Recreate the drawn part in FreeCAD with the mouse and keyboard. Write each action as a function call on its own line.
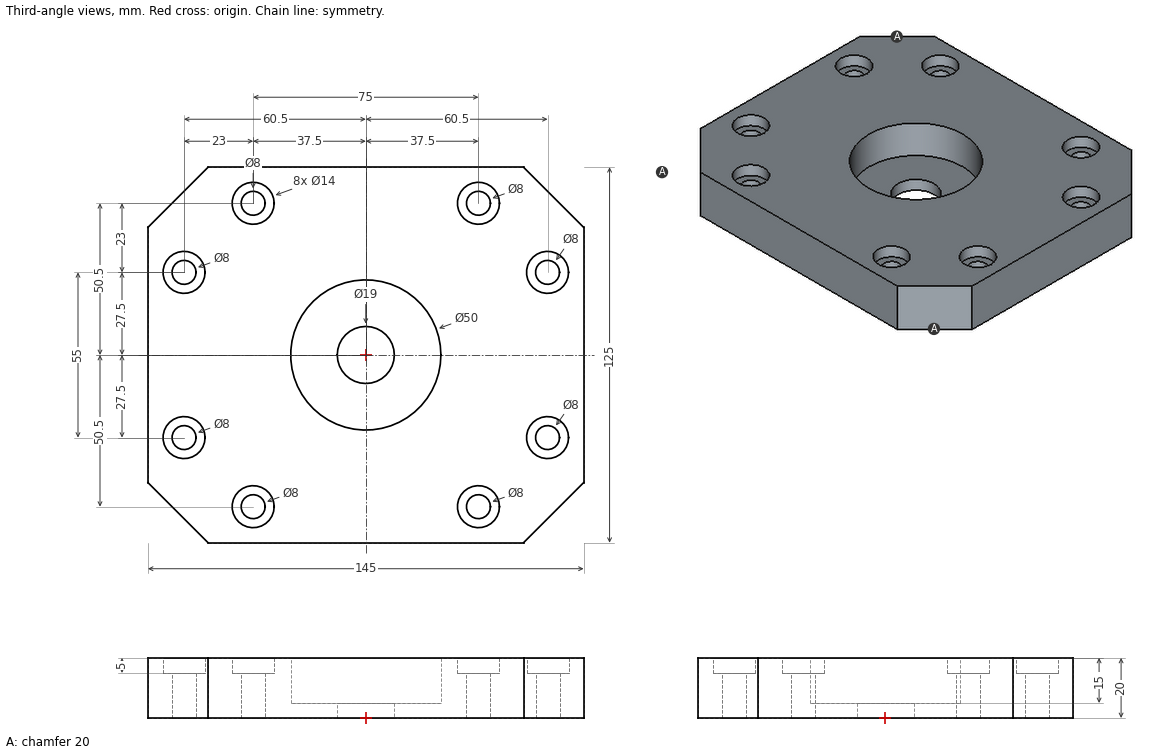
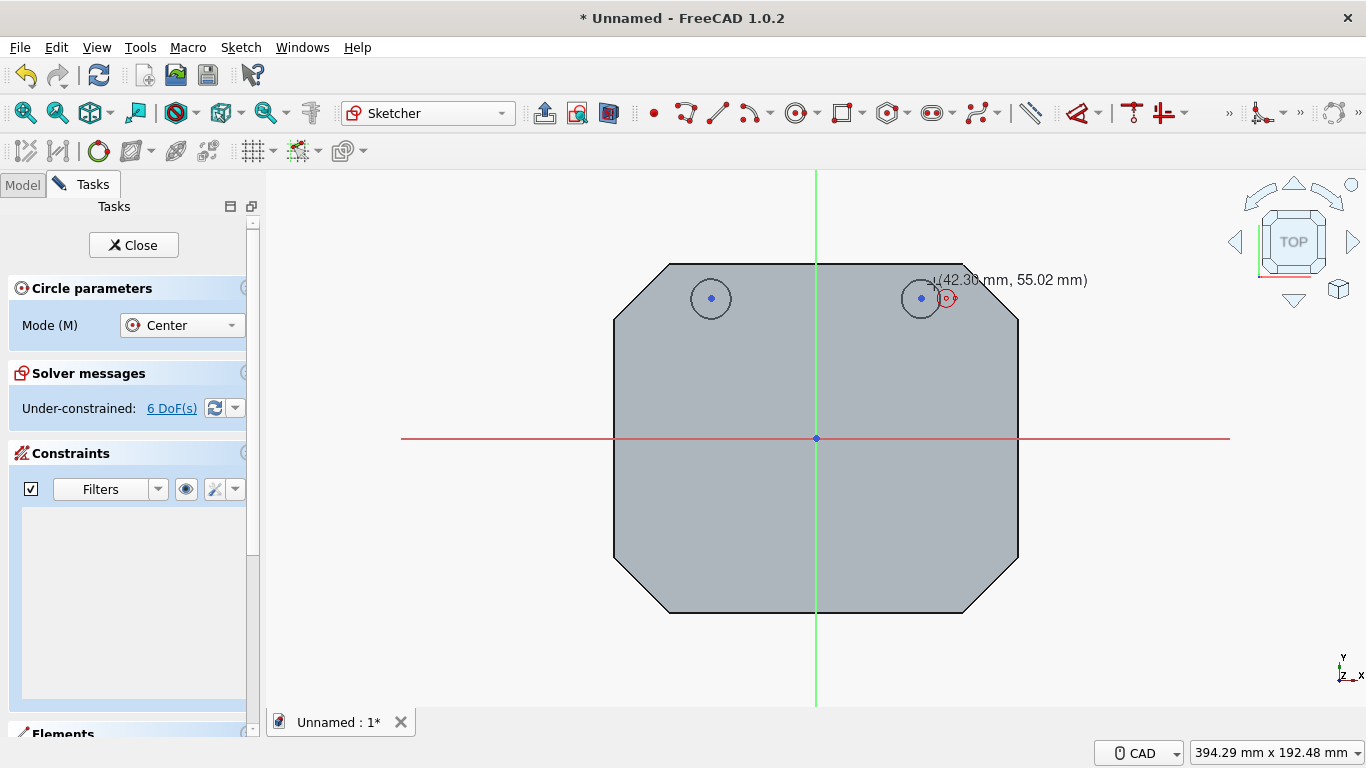
click(647, 362)
click(661, 348)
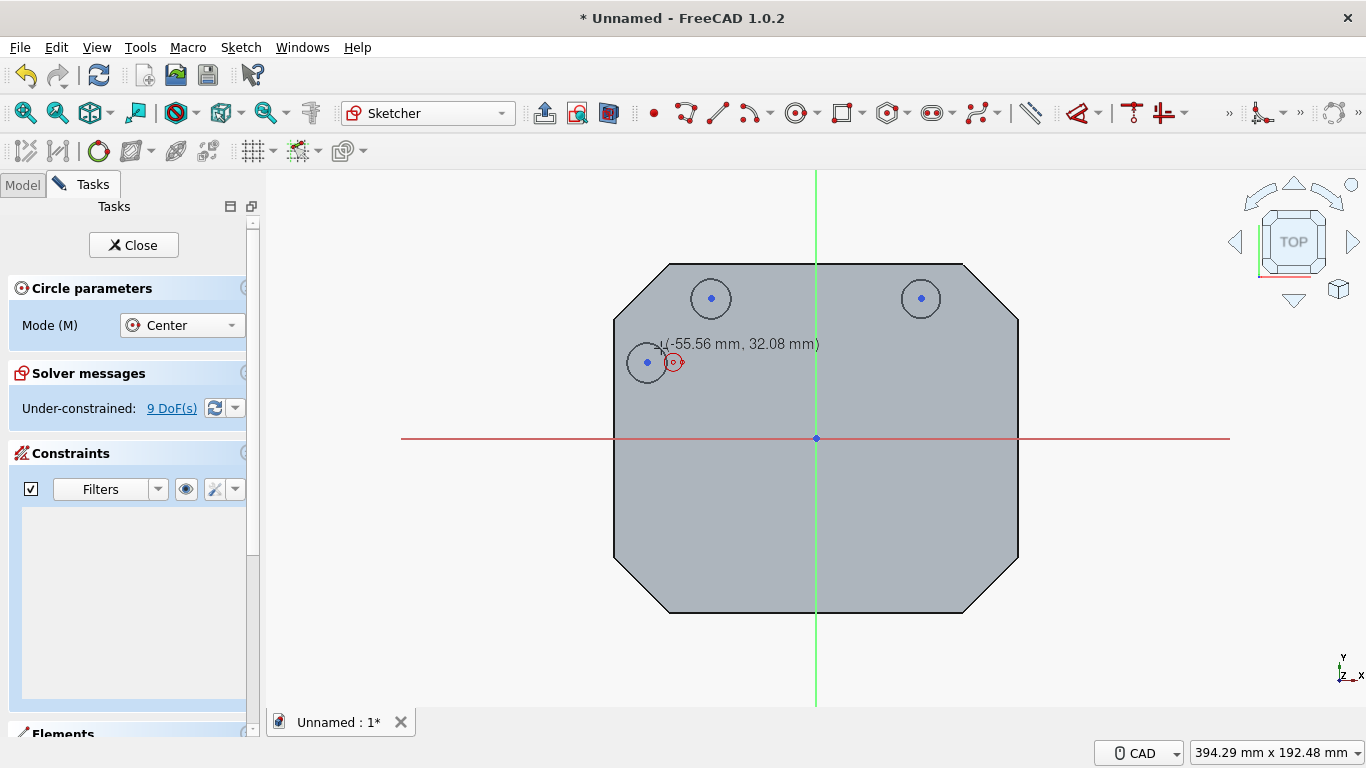
click(647, 515)
click(661, 501)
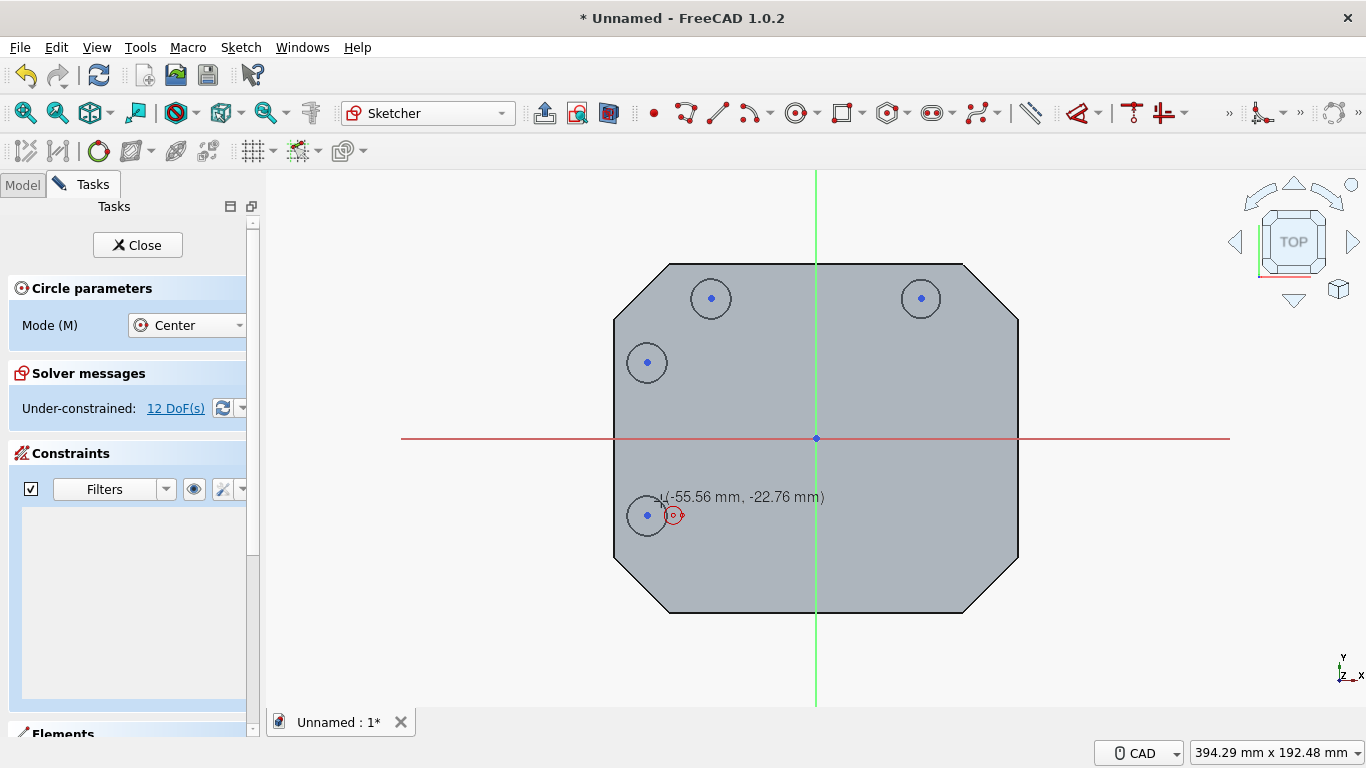
click(711, 579)
click(725, 566)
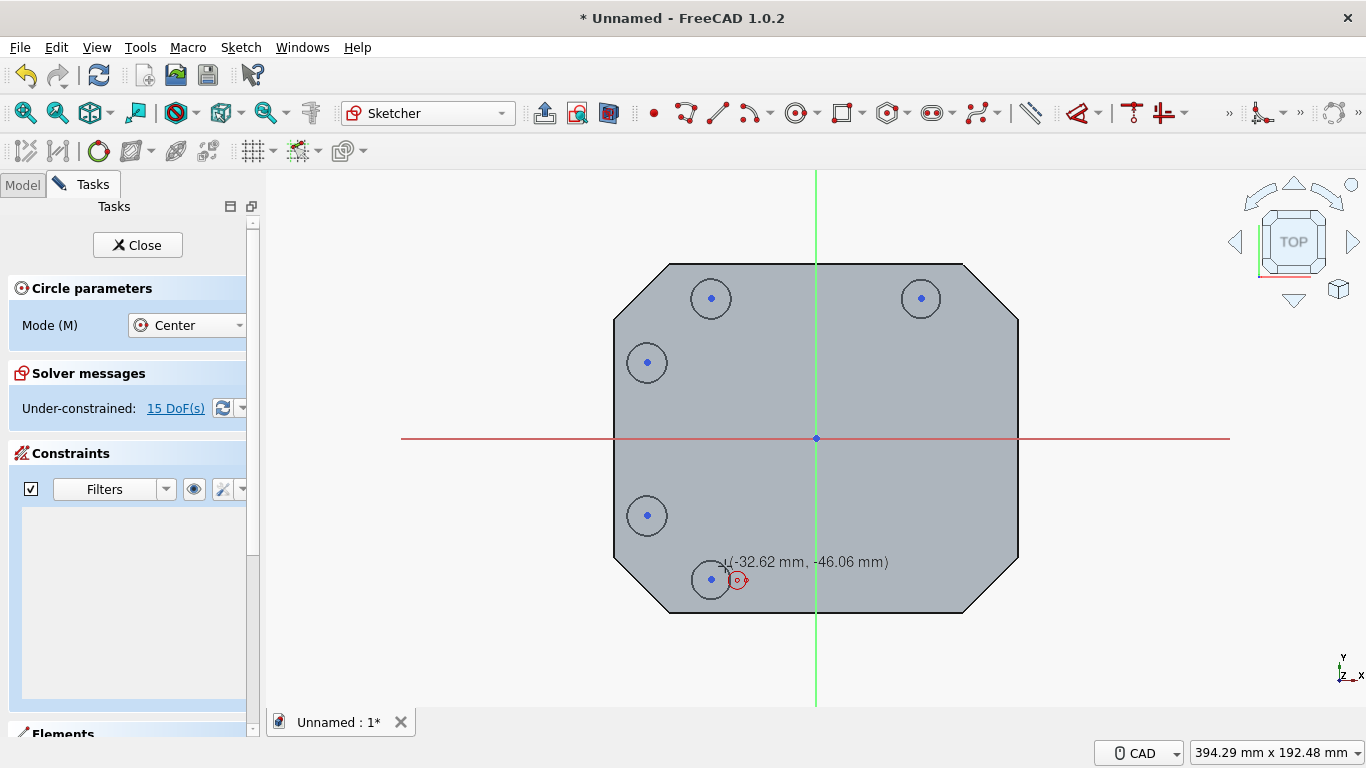
click(921, 579)
click(934, 566)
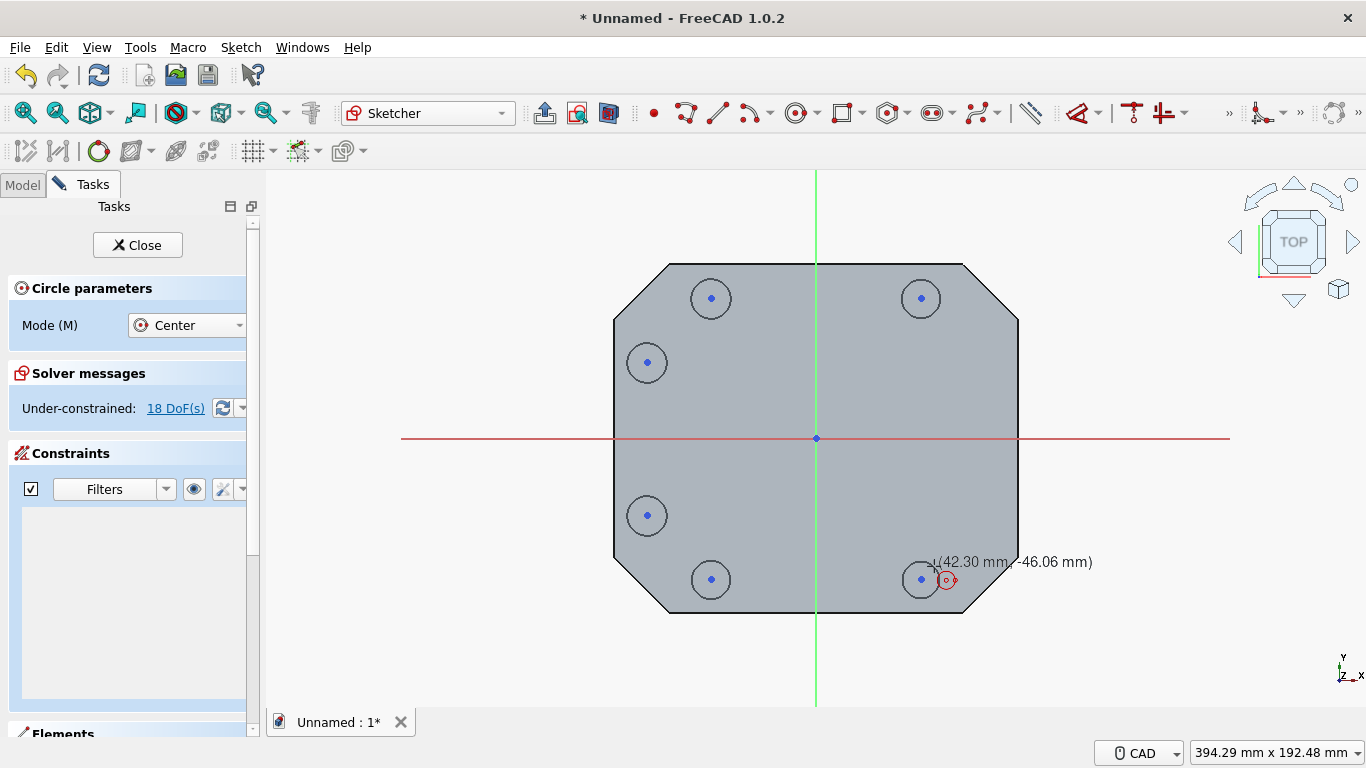
click(985, 362)
click(999, 348)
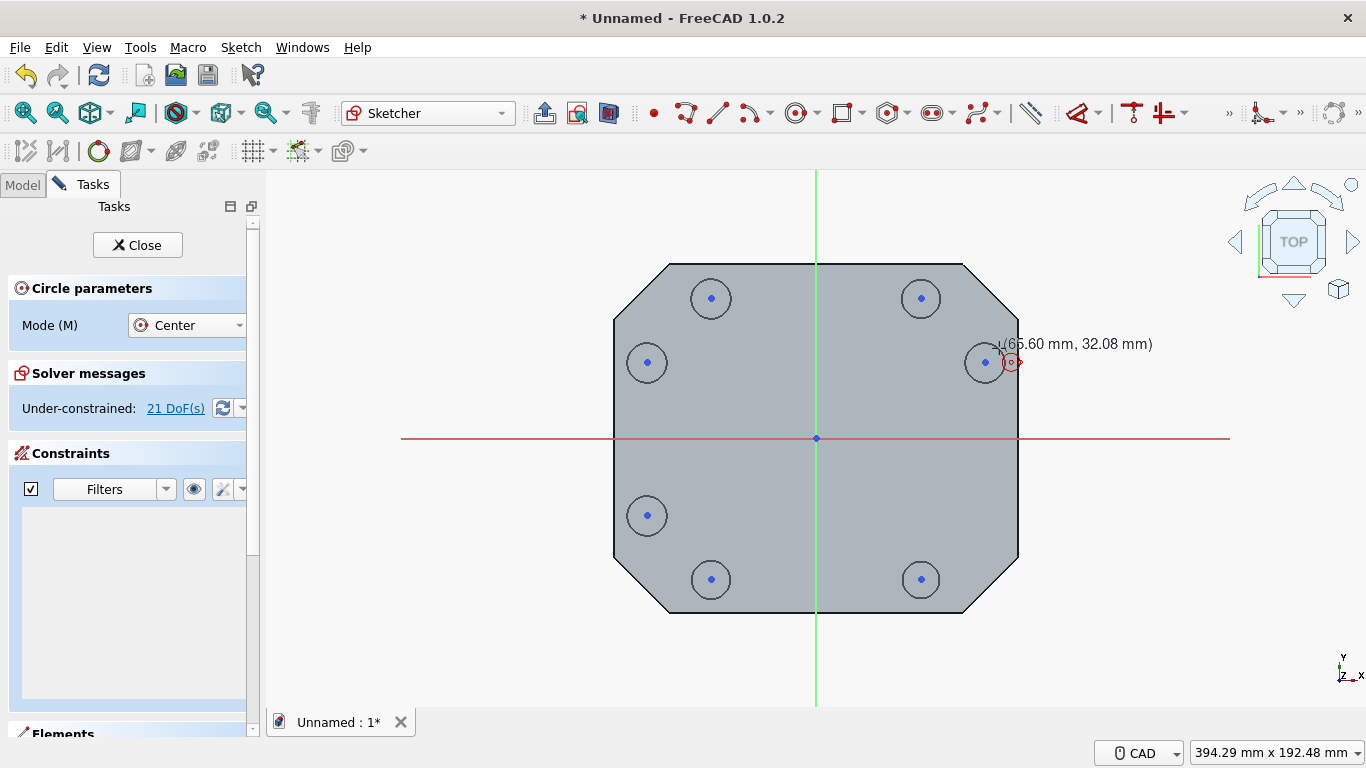
click(985, 515)
click(999, 501)
key(Escape)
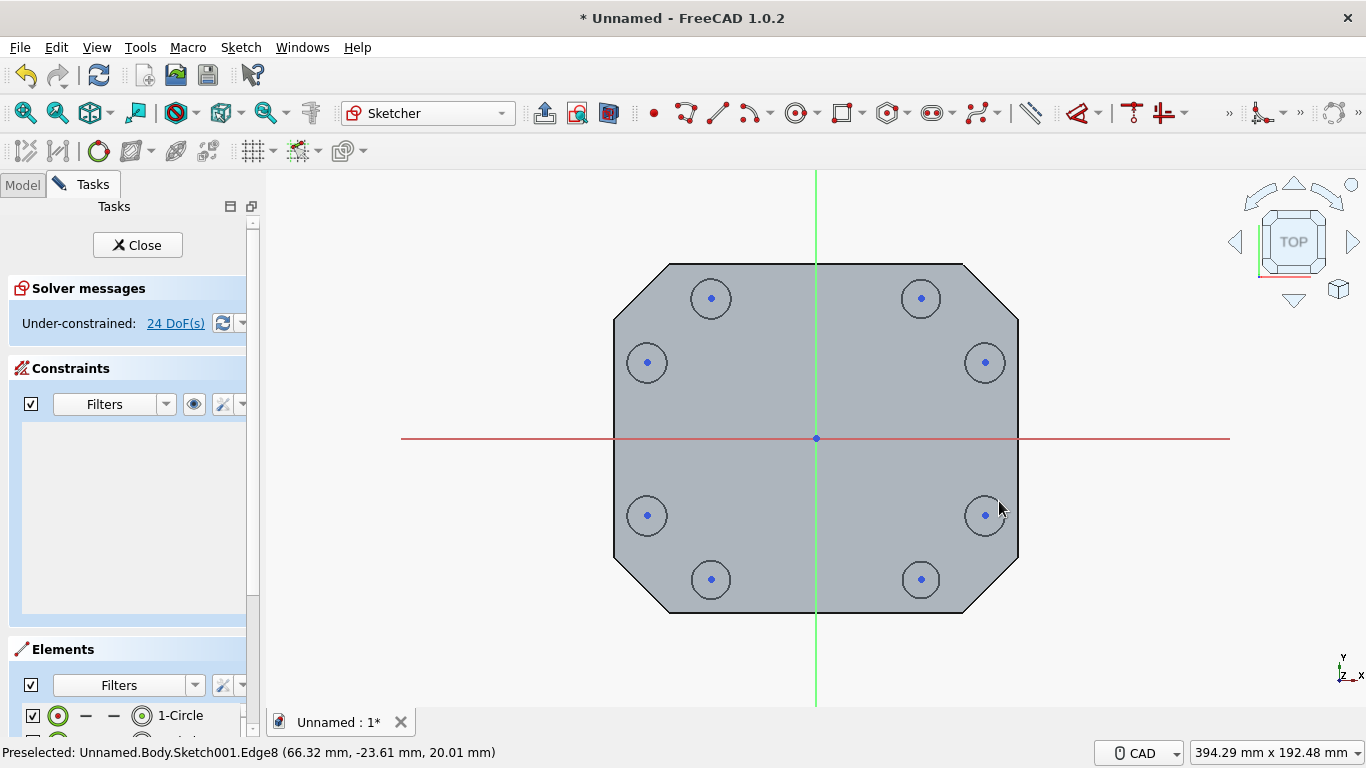
click(725, 285)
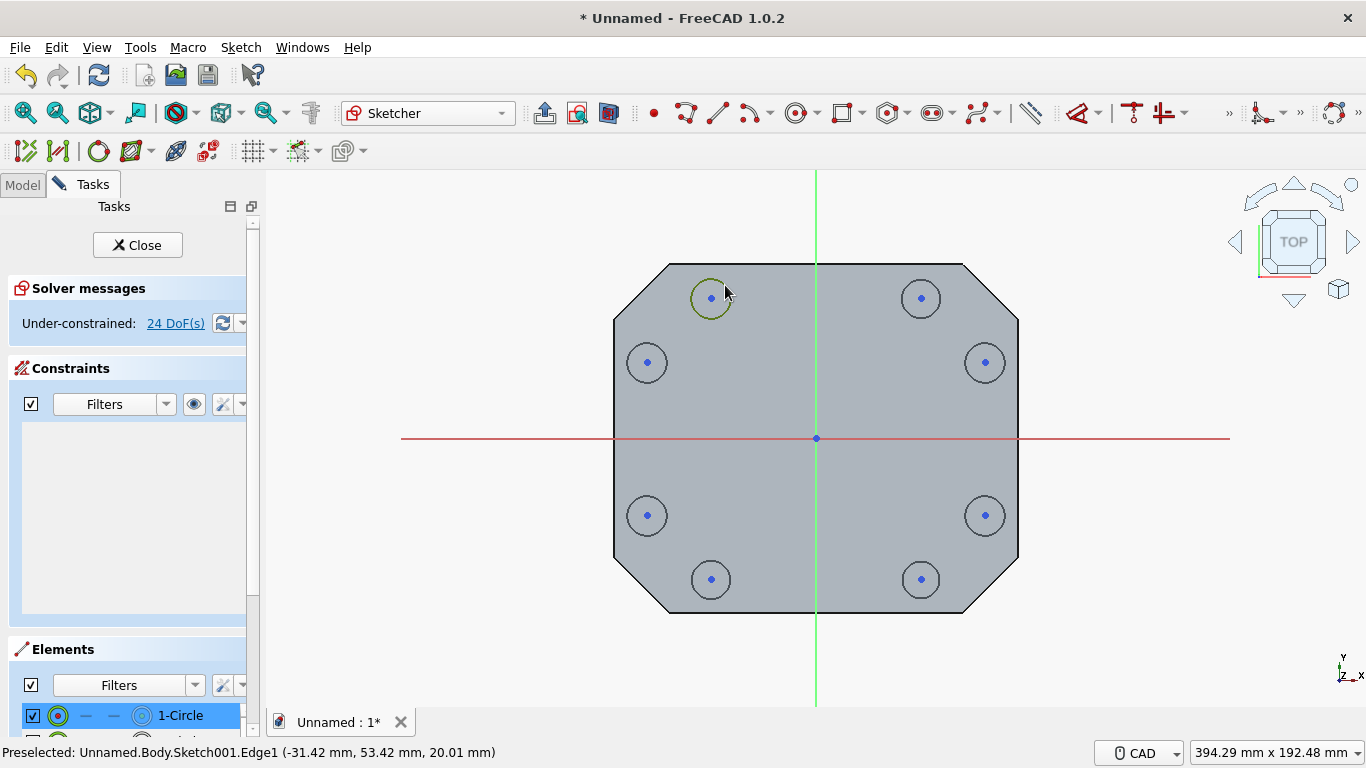
click(934, 285)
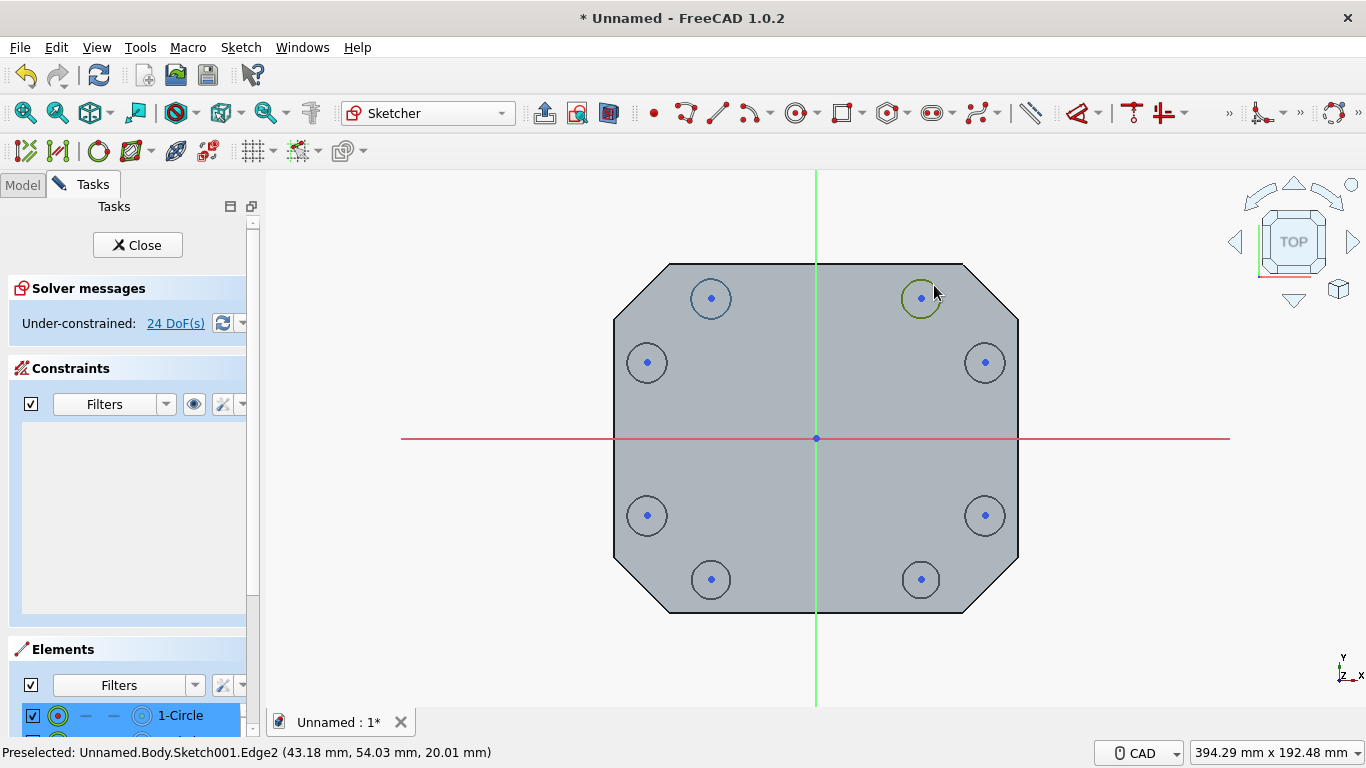
click(661, 349)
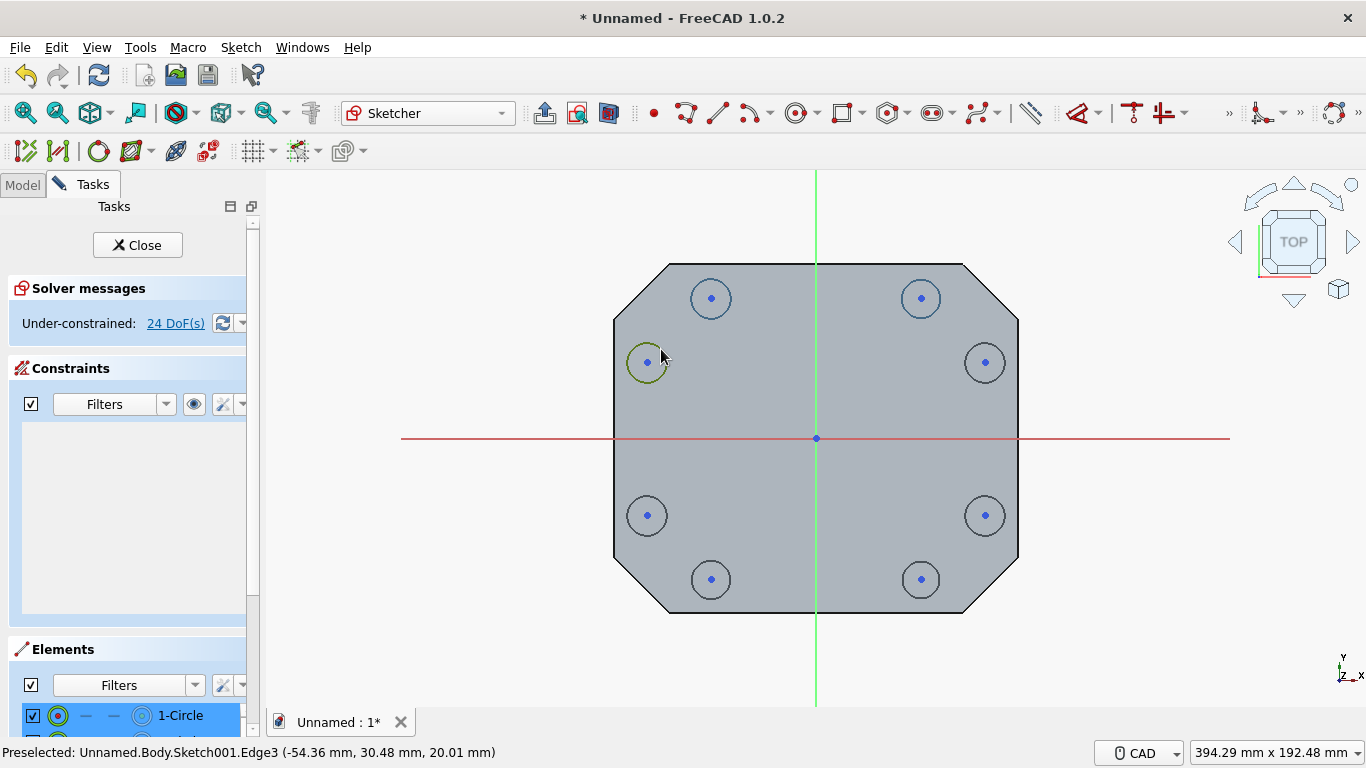
click(661, 502)